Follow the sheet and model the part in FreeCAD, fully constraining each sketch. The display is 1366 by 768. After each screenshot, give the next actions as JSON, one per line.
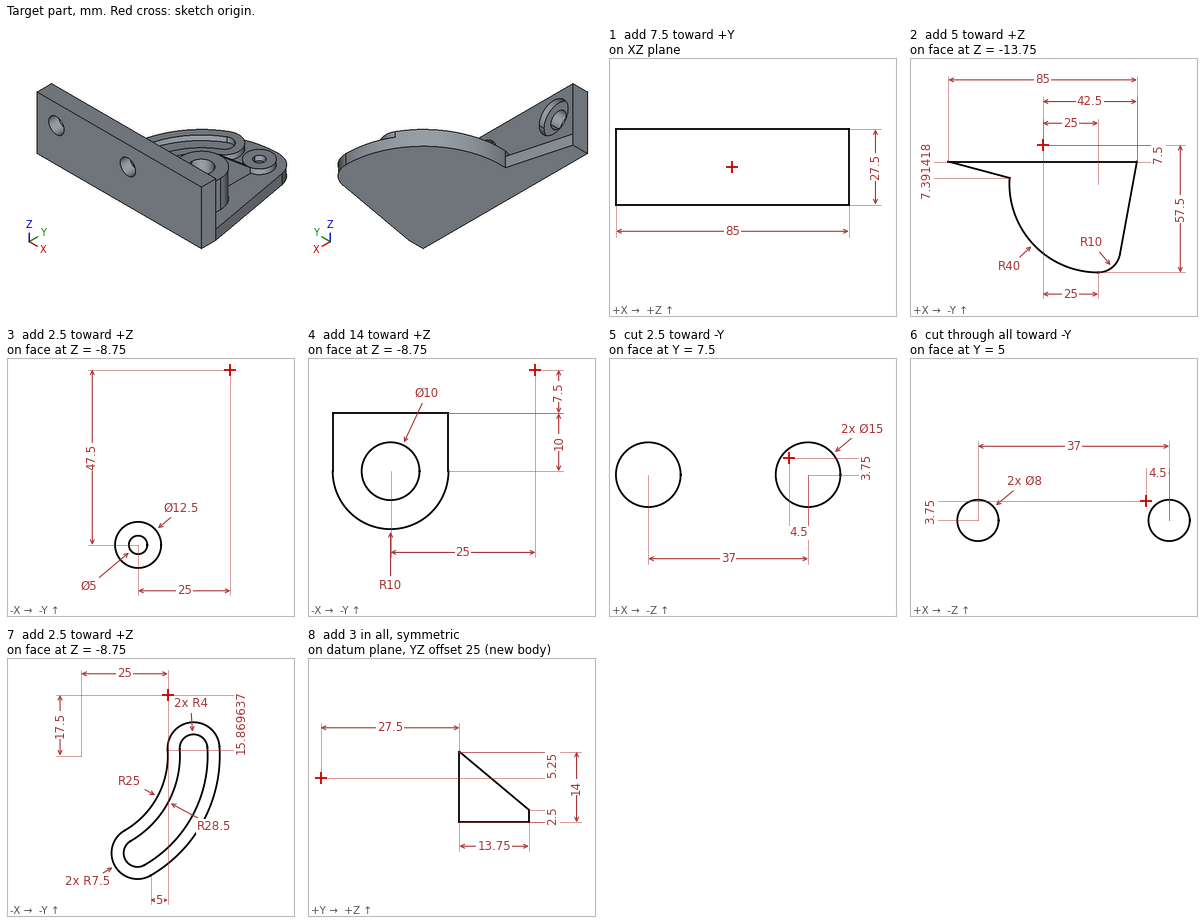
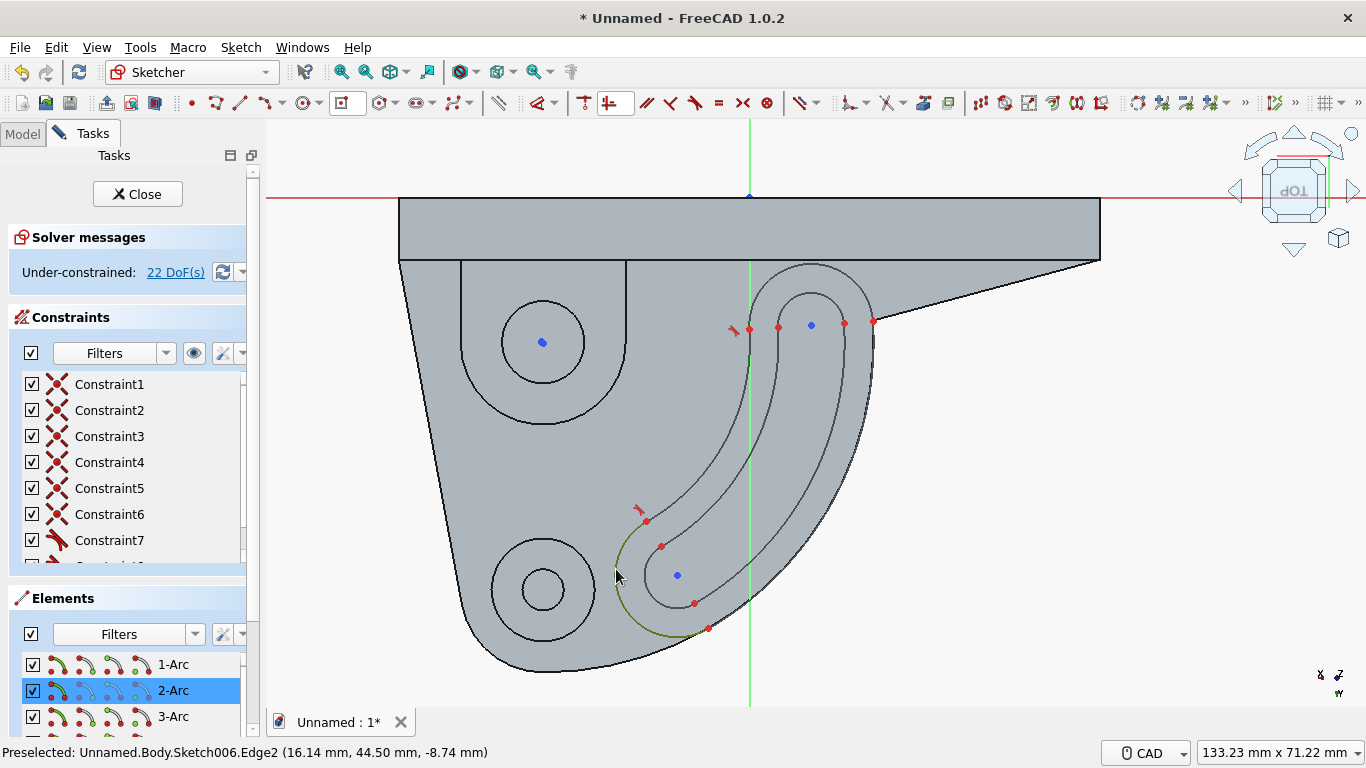
{"action": "left_click", "coordinate": [792, 559]}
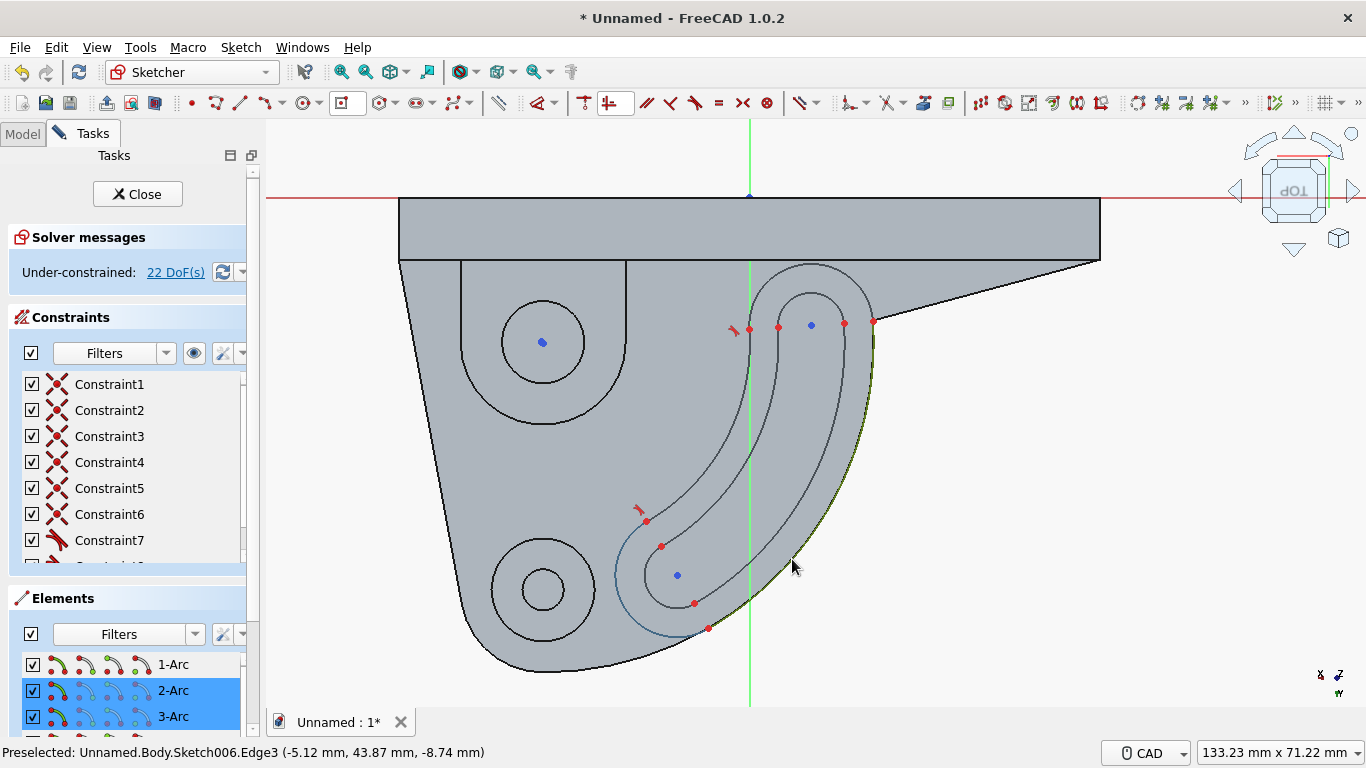
{"action": "left_click", "coordinate": [696, 104]}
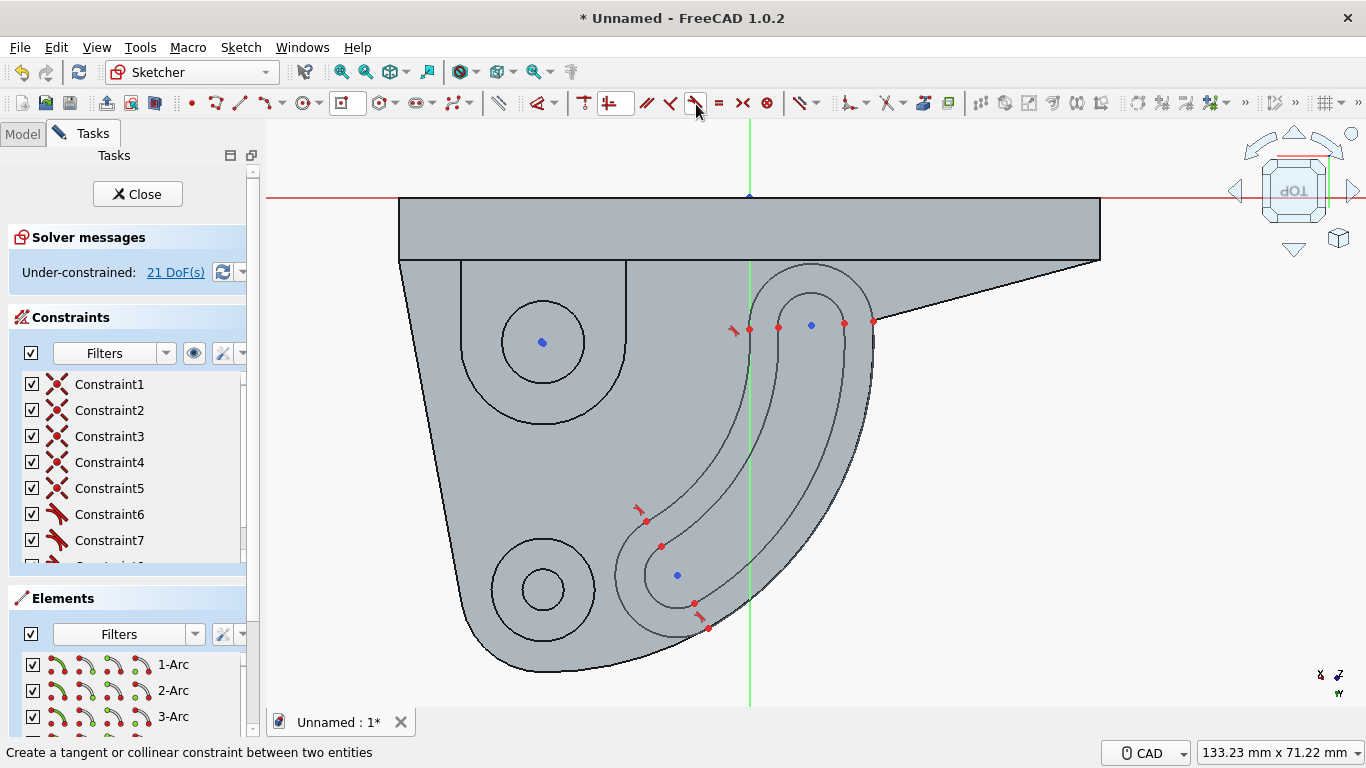
{"action": "left_click", "coordinate": [792, 559]}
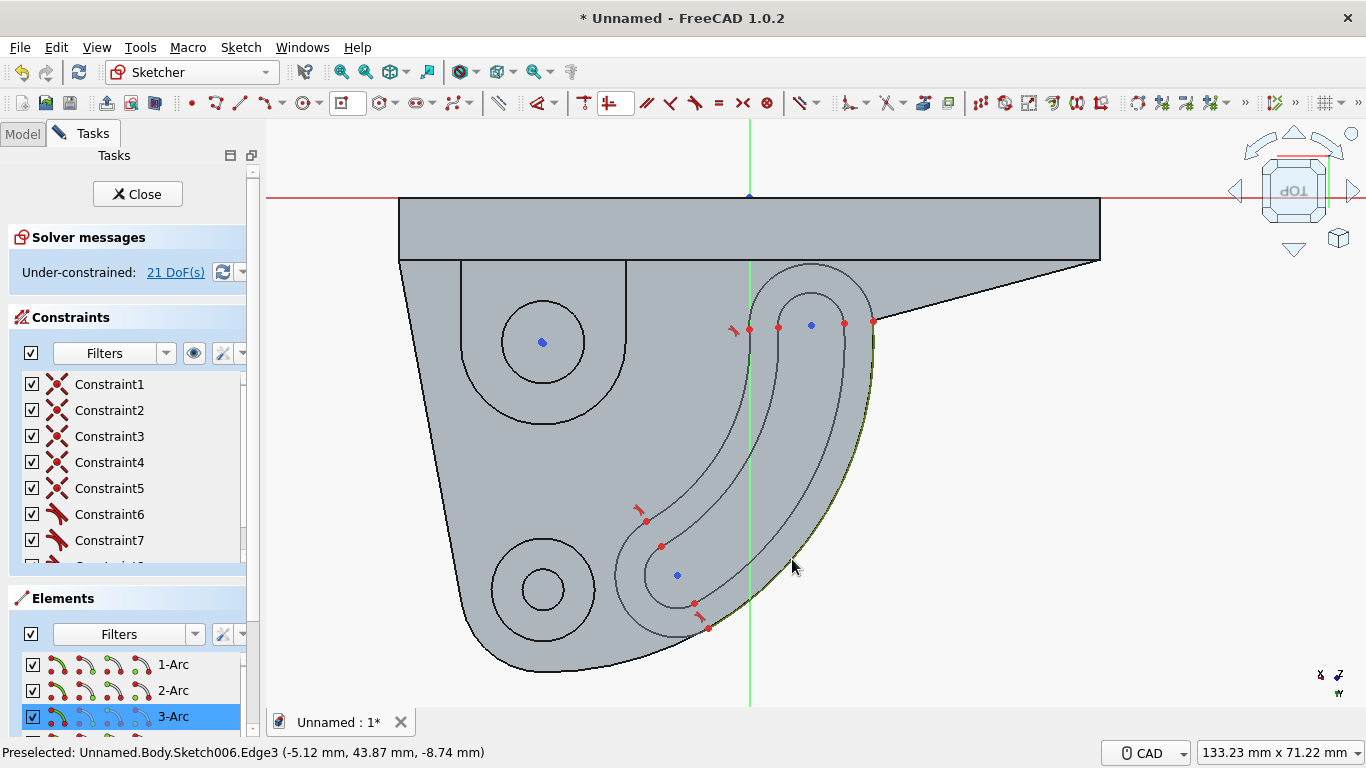
{"action": "left_click", "coordinate": [844, 274]}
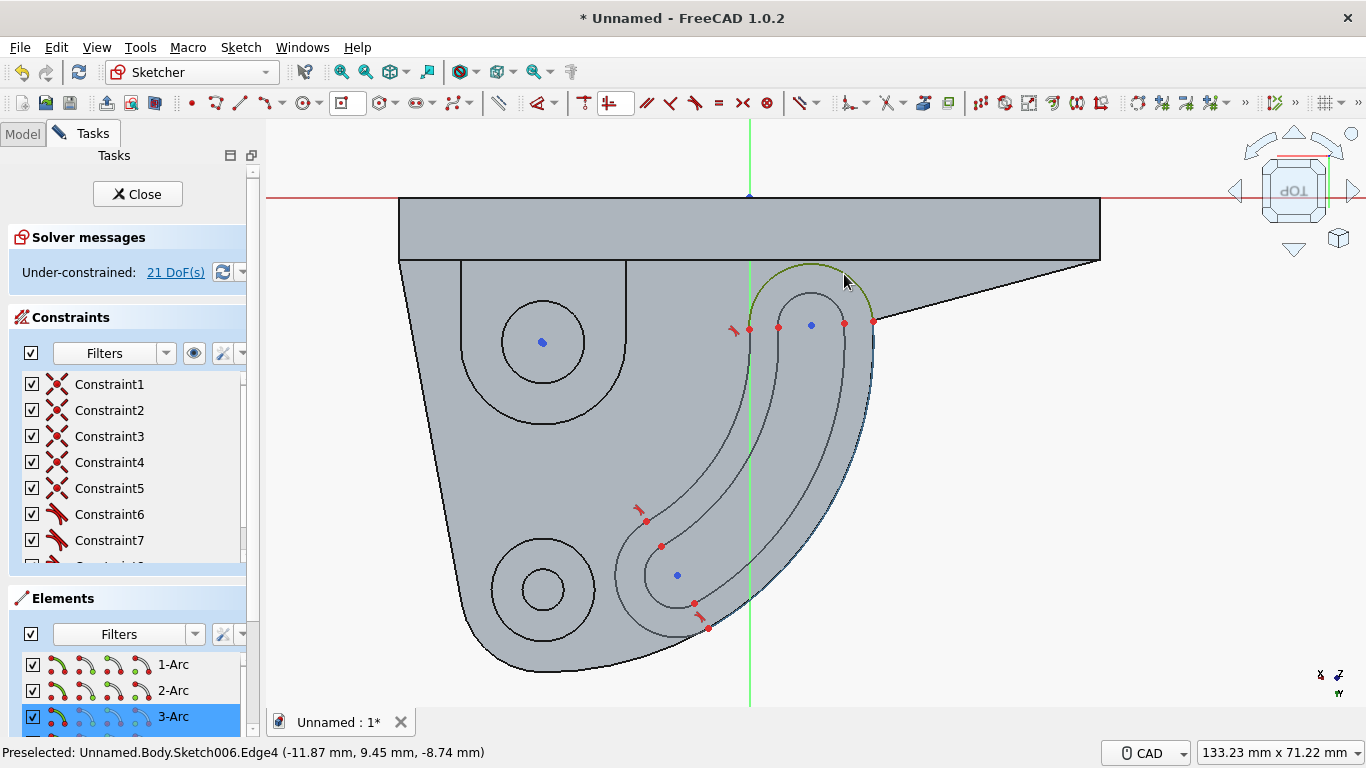
{"action": "left_click", "coordinate": [696, 104]}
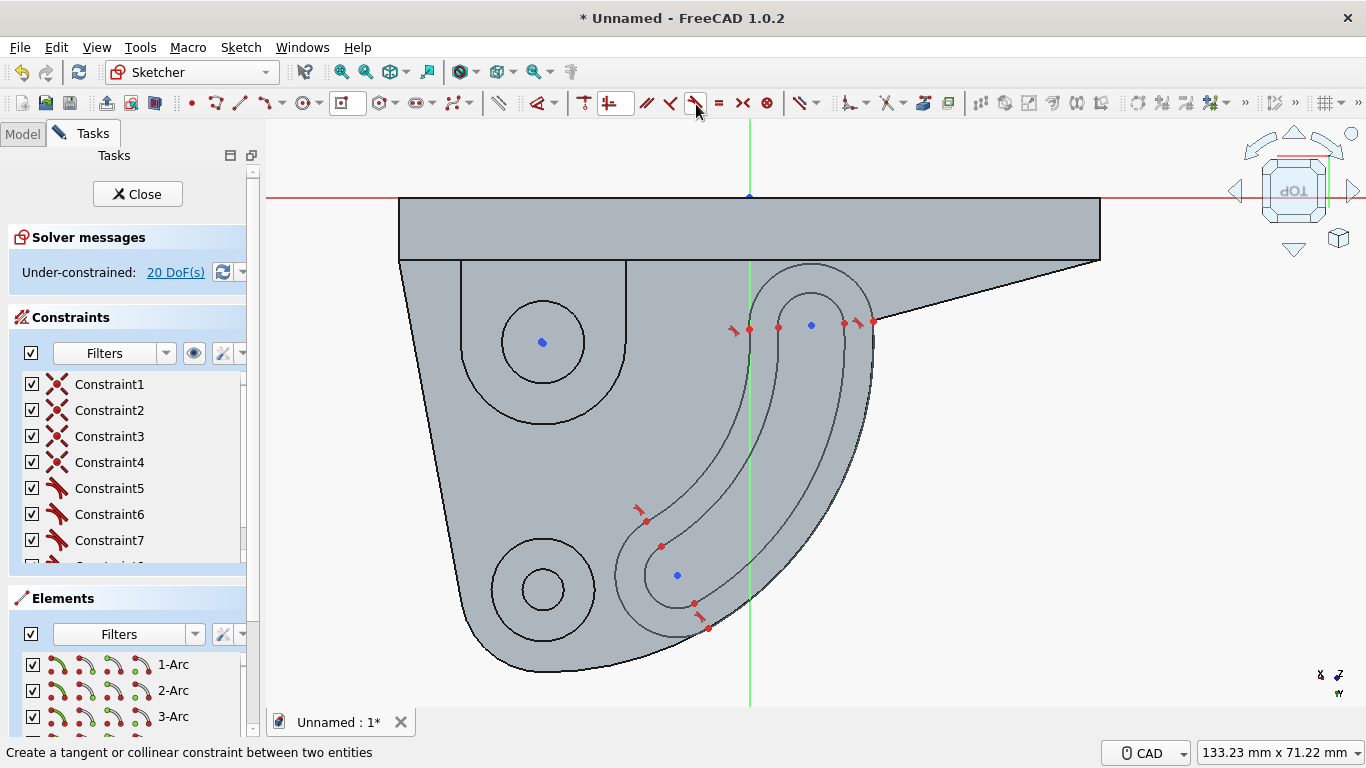
{"action": "left_click", "coordinate": [829, 298]}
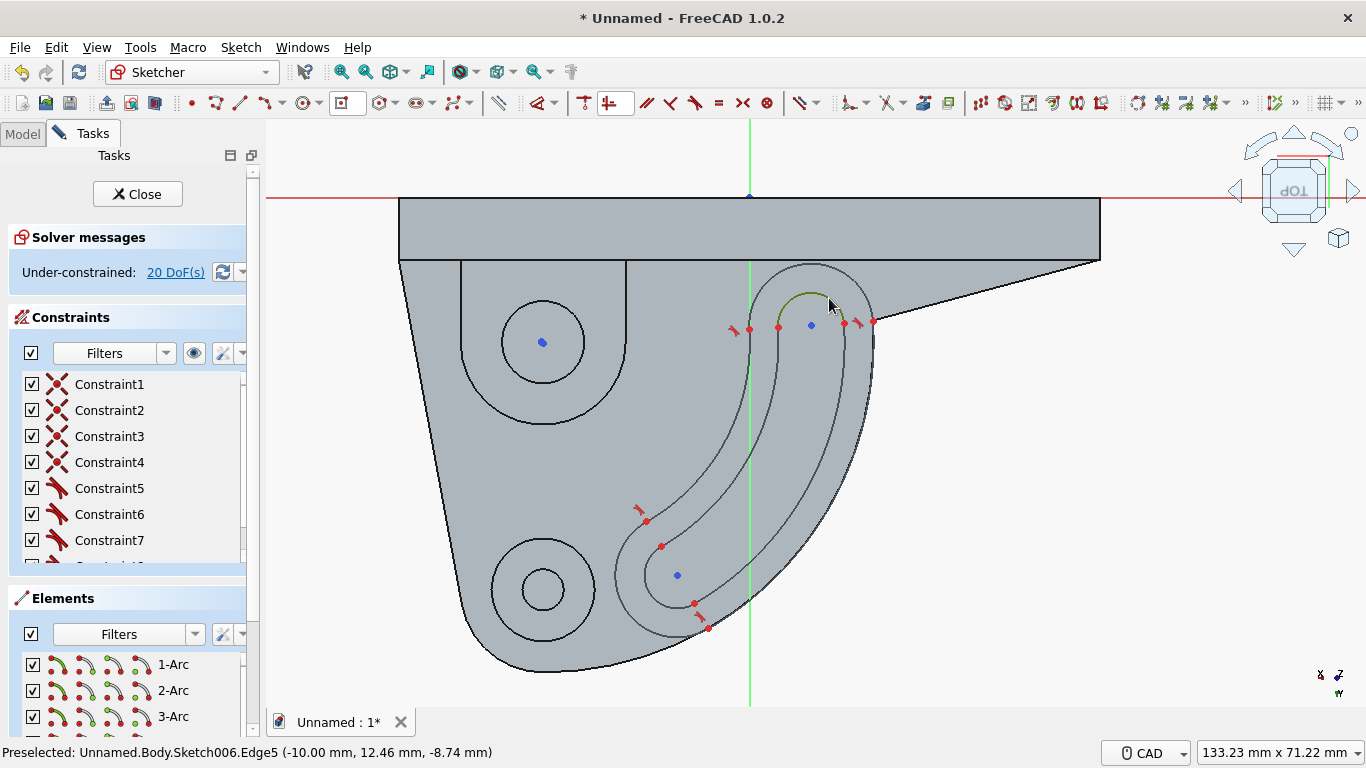
{"action": "left_click", "coordinate": [771, 540]}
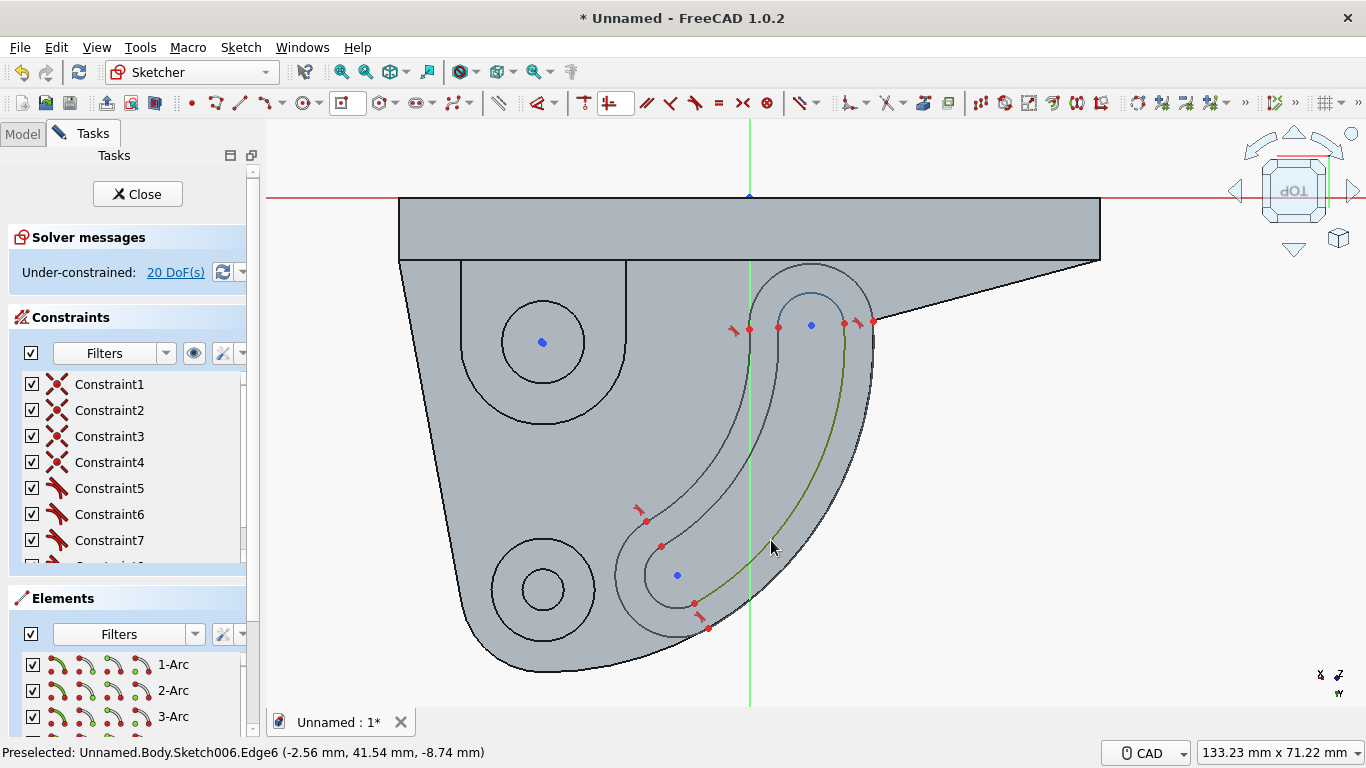
{"action": "left_click", "coordinate": [696, 104]}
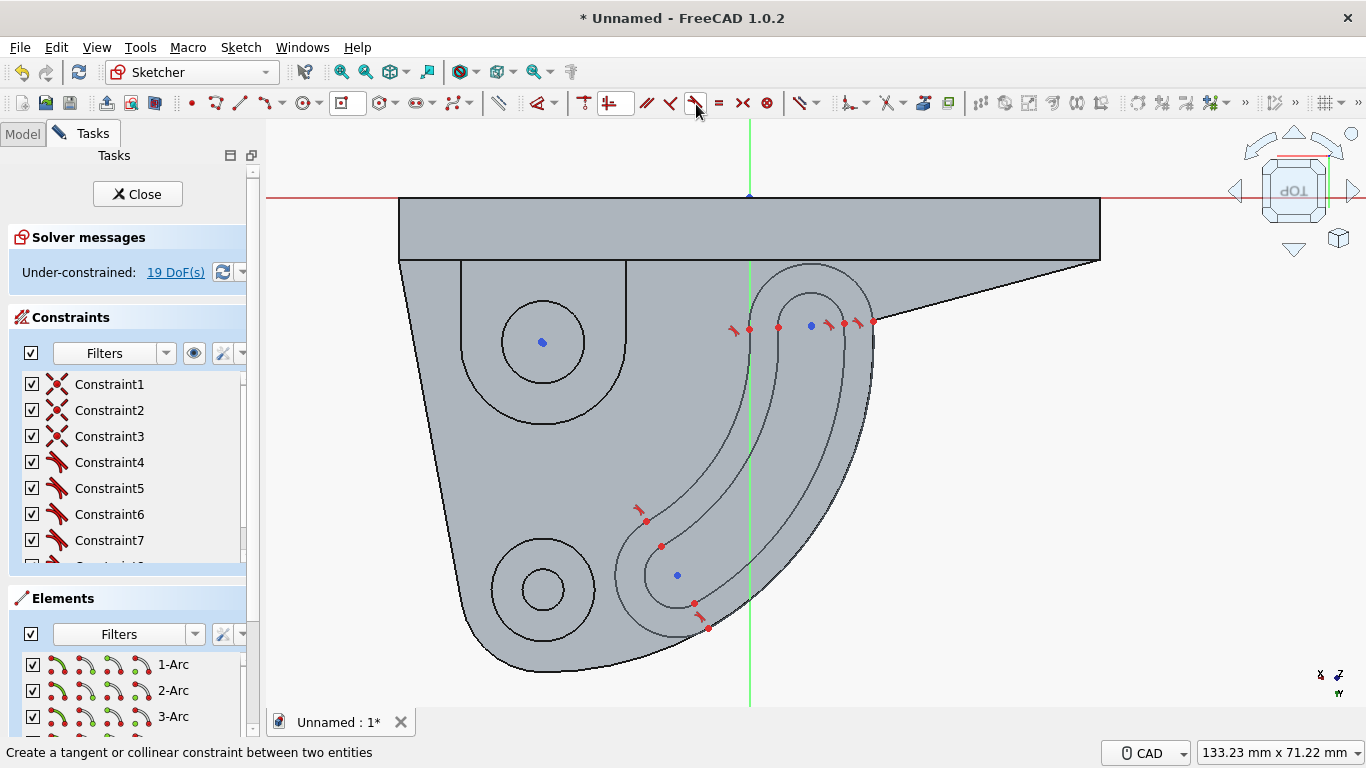
{"action": "left_click", "coordinate": [829, 298]}